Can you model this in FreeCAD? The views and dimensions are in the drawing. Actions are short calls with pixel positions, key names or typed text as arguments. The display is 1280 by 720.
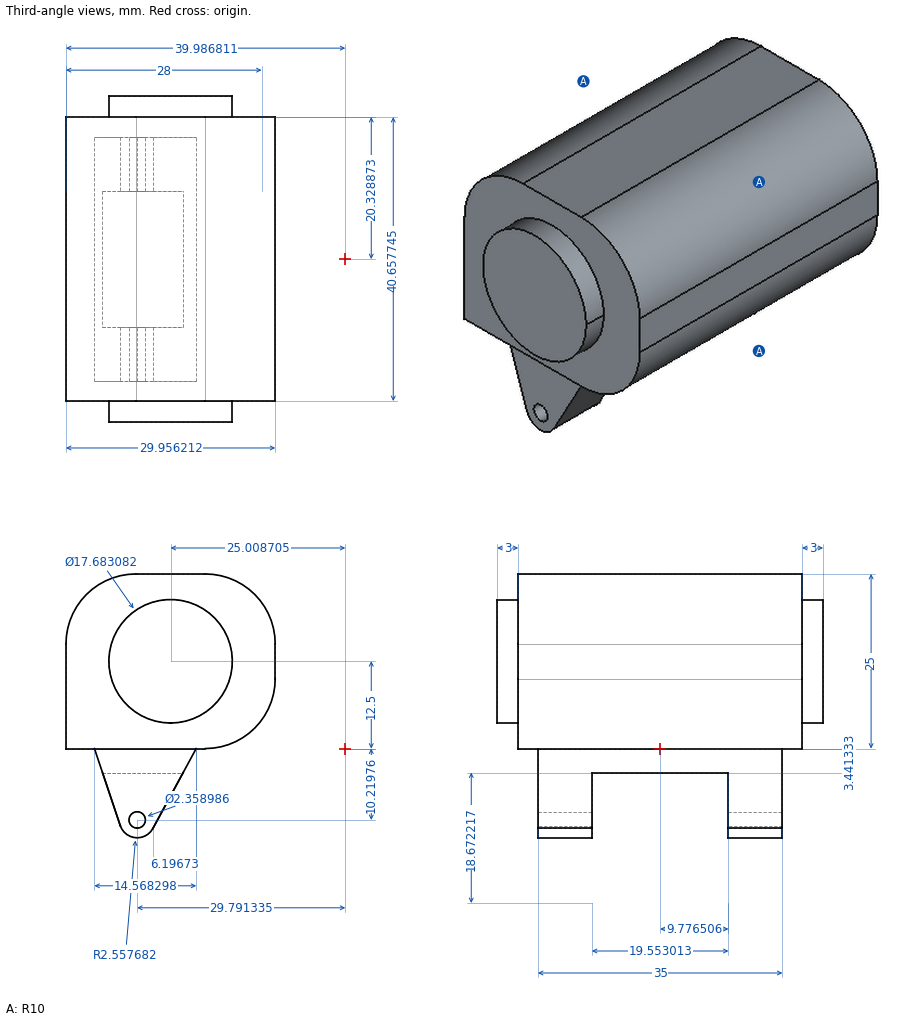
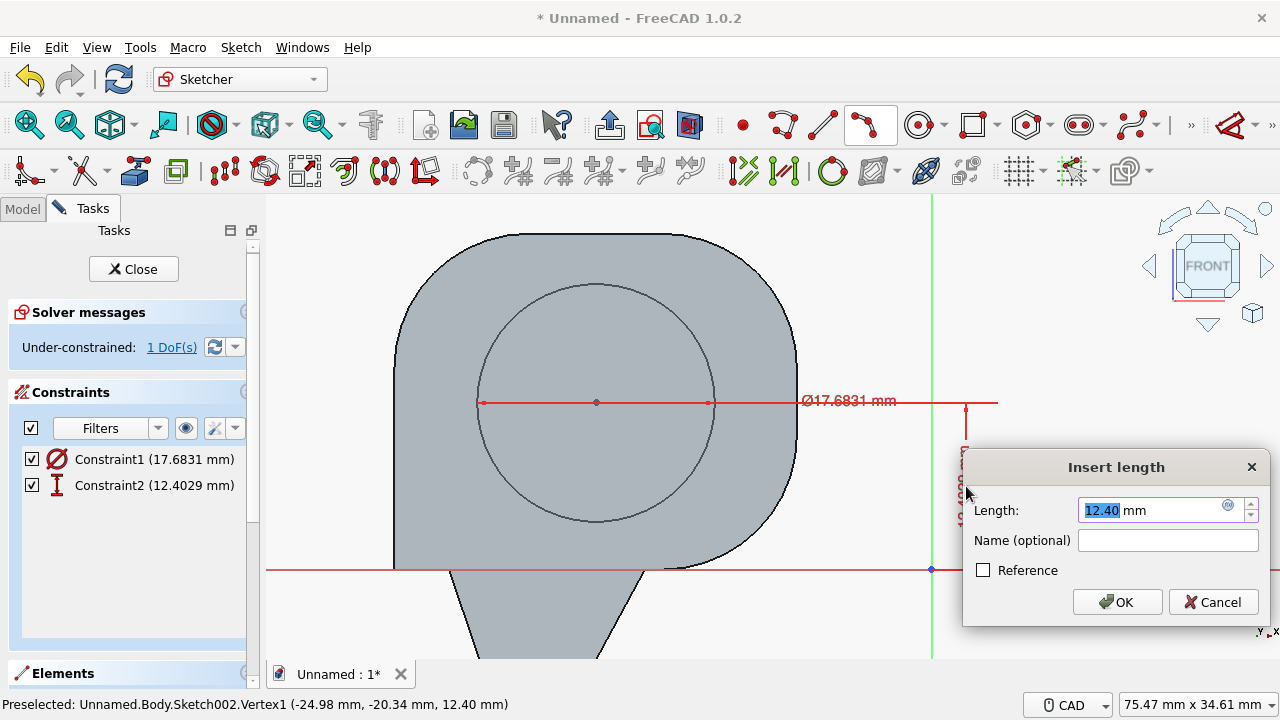
text(12.5)
key(Return)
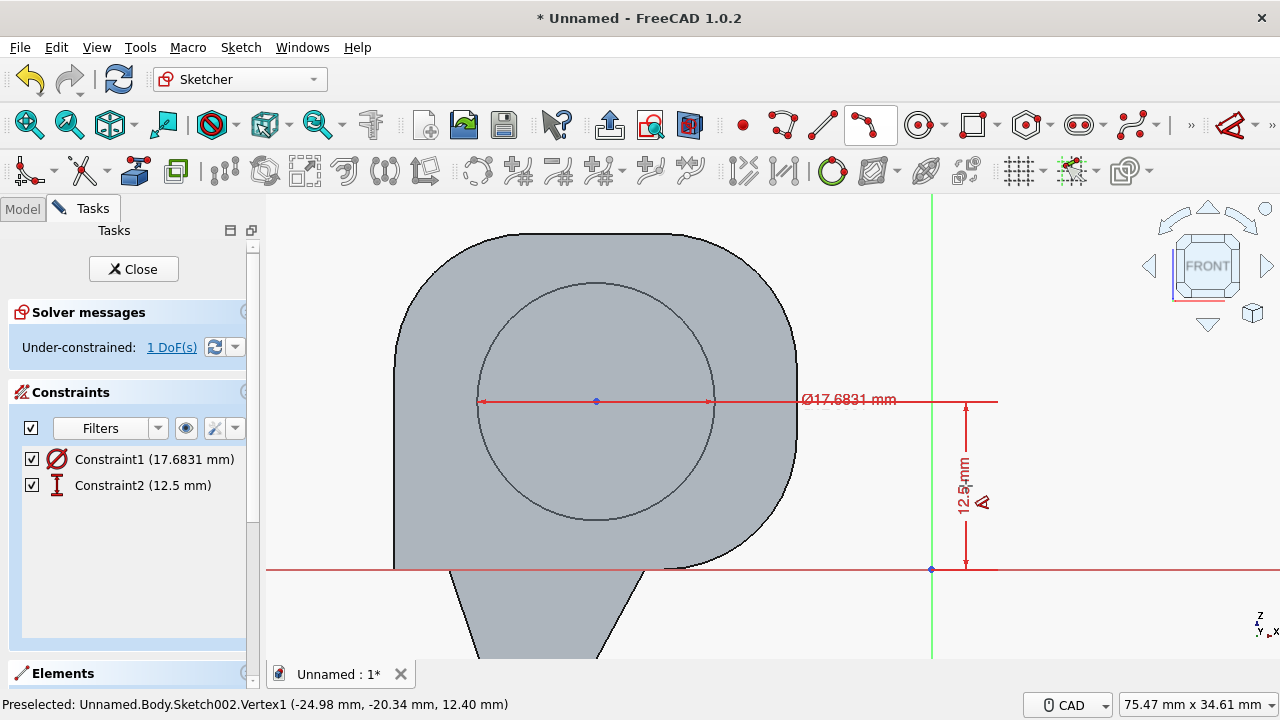
click(596, 402)
click(764, 604)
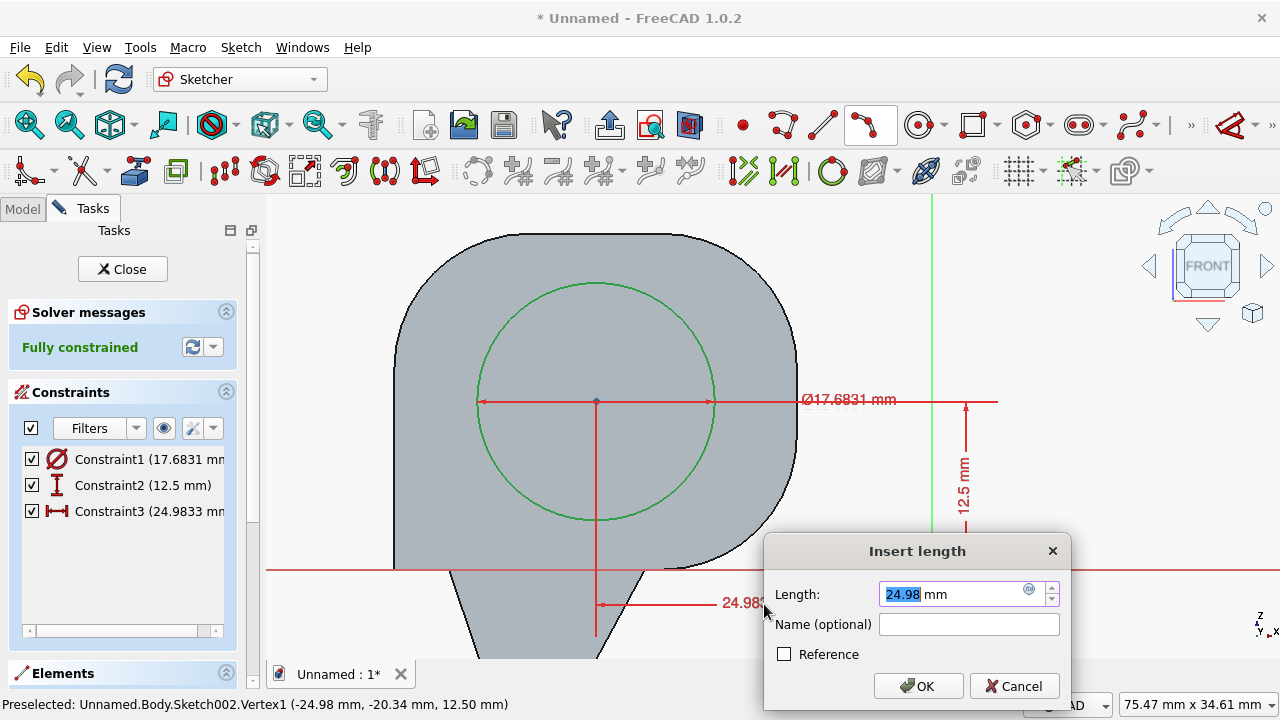
text(25.008705)
key(Return)
key(Escape)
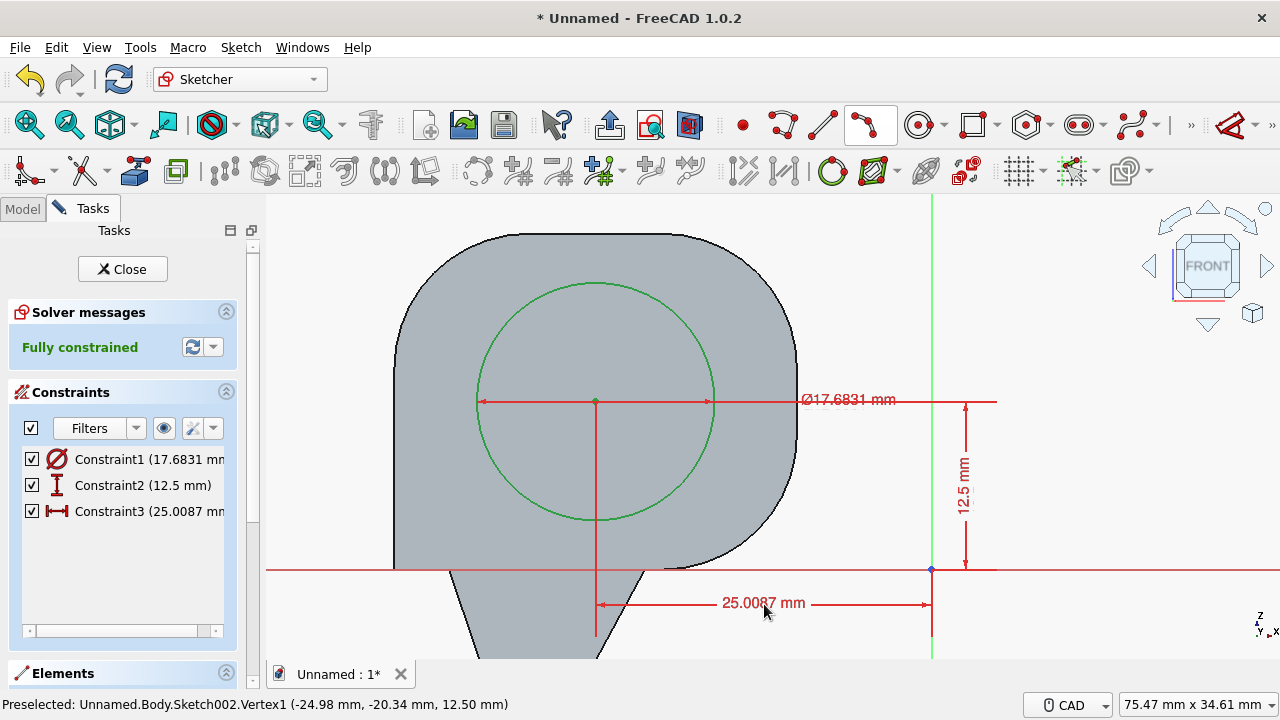
click(123, 269)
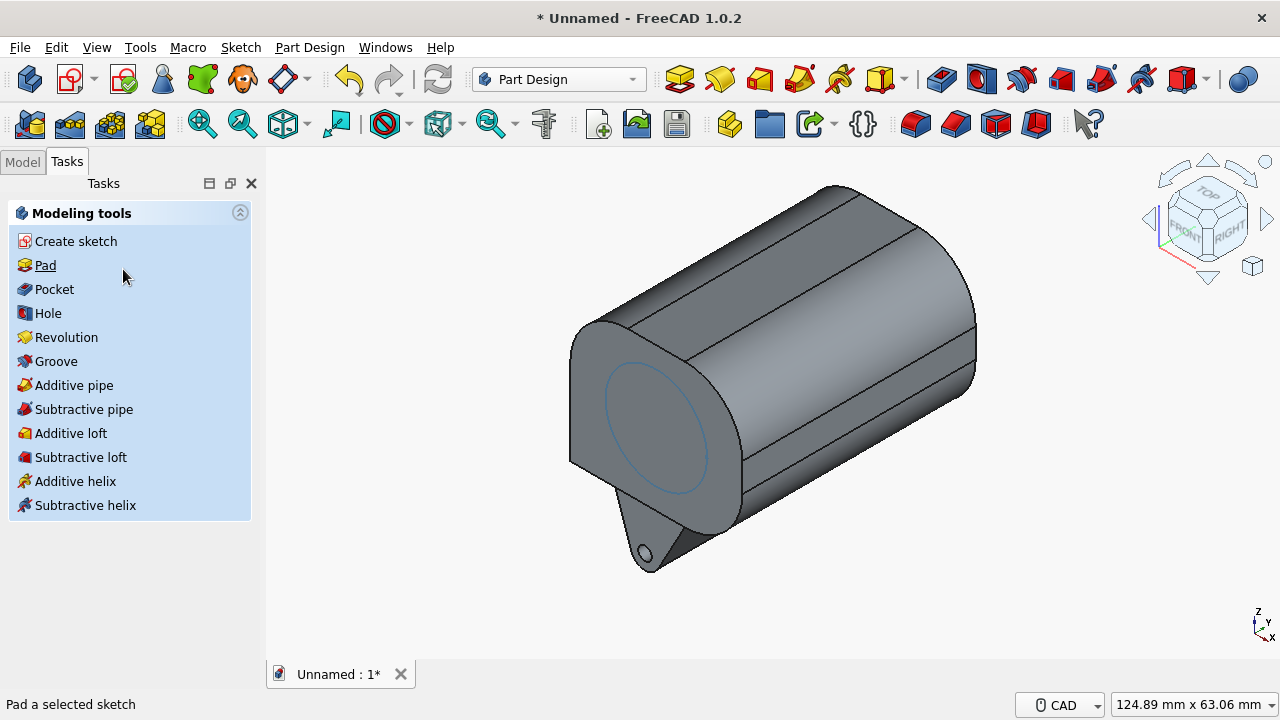
click(680, 80)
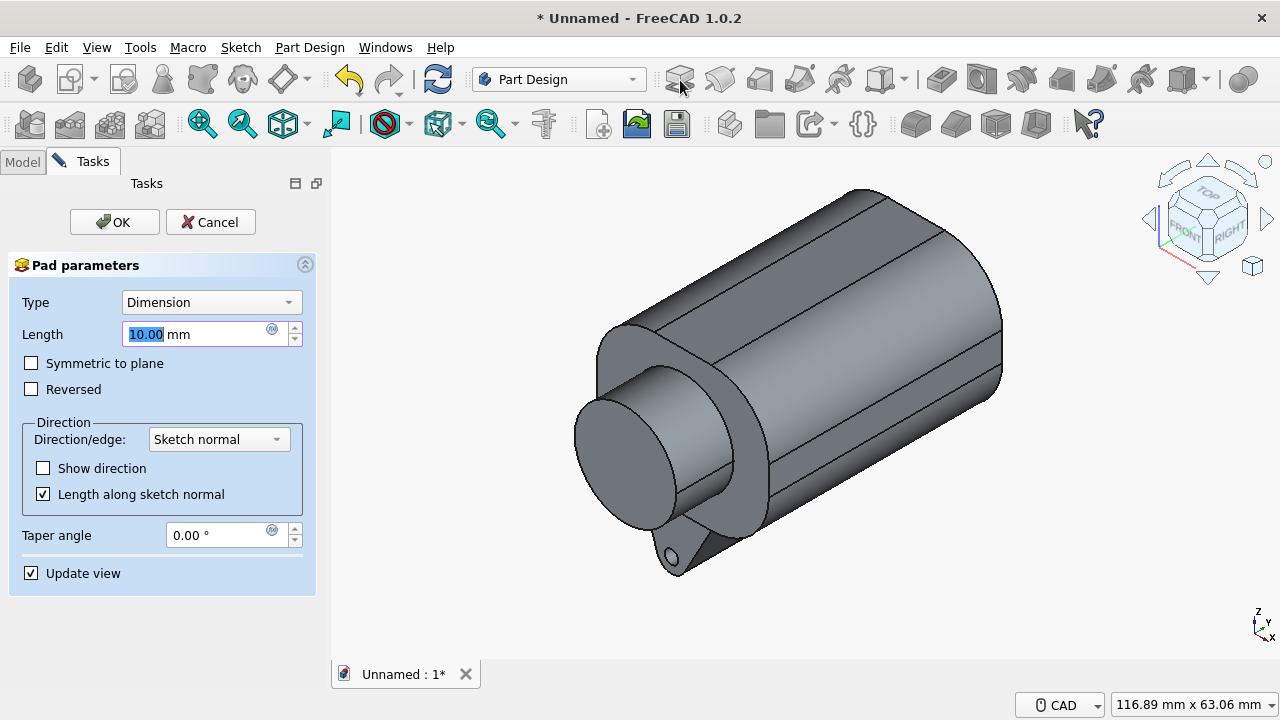
text(3)
key(Tab)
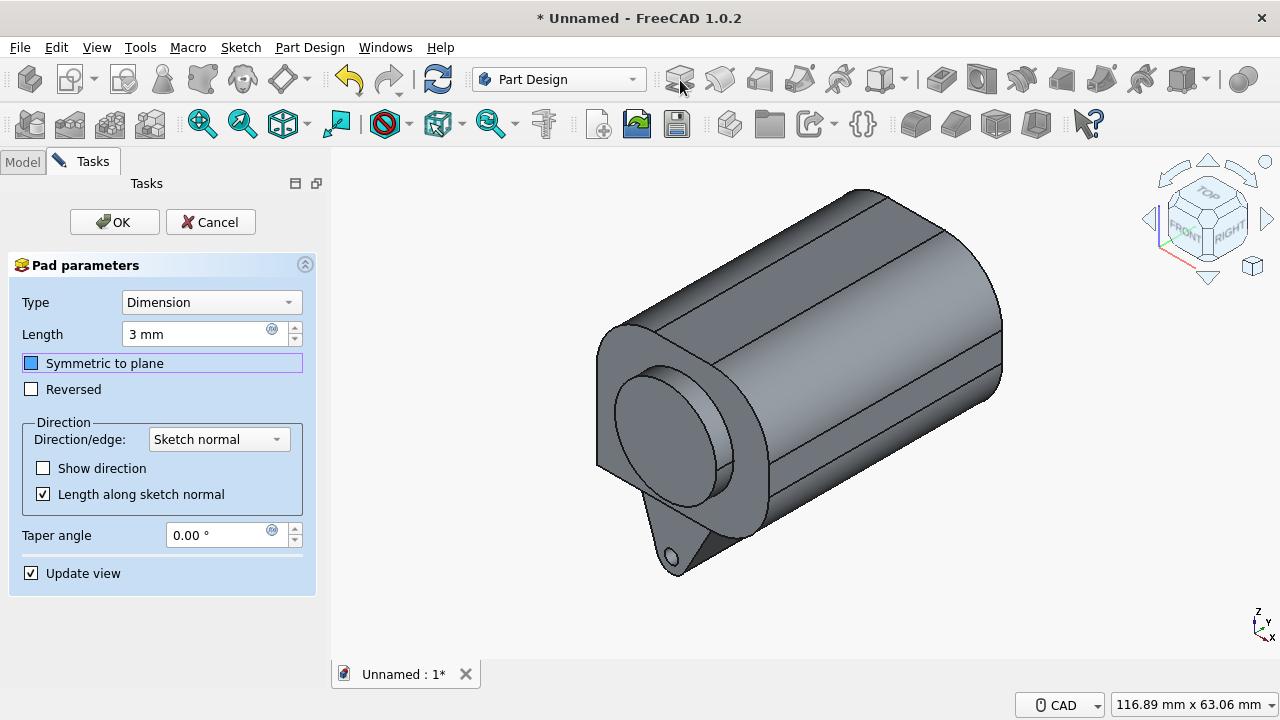
click(115, 222)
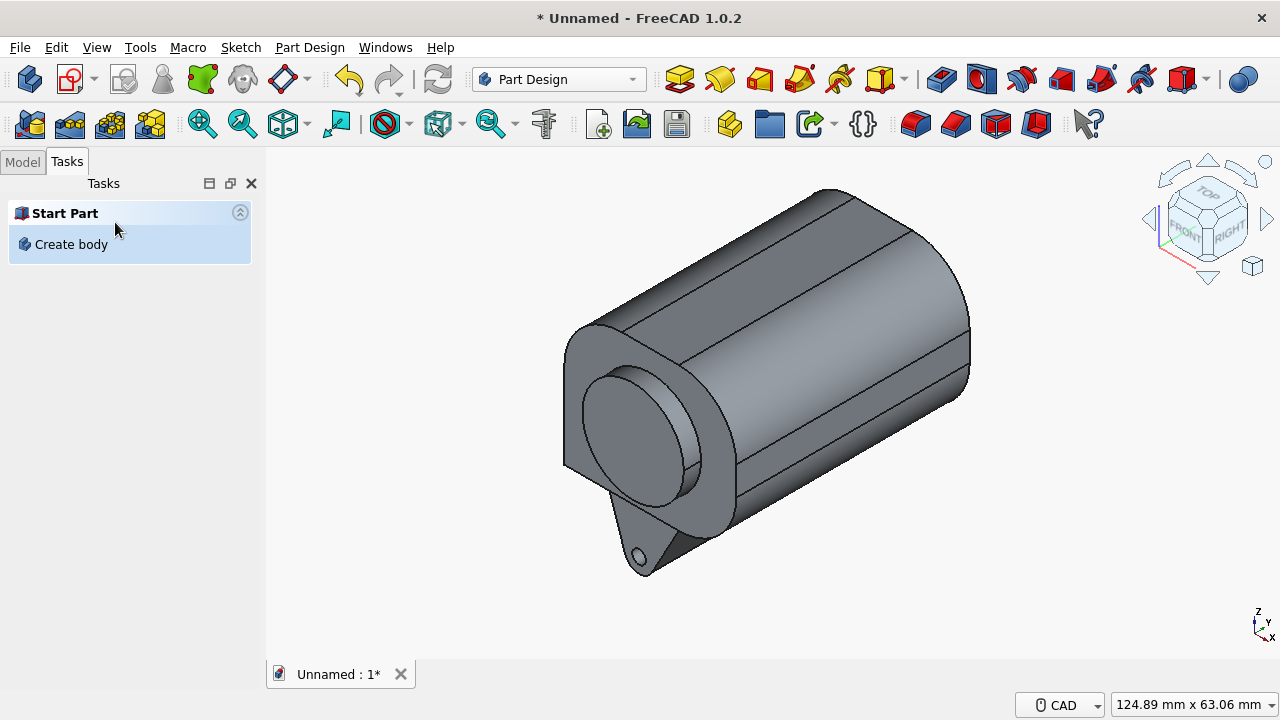
click(23, 161)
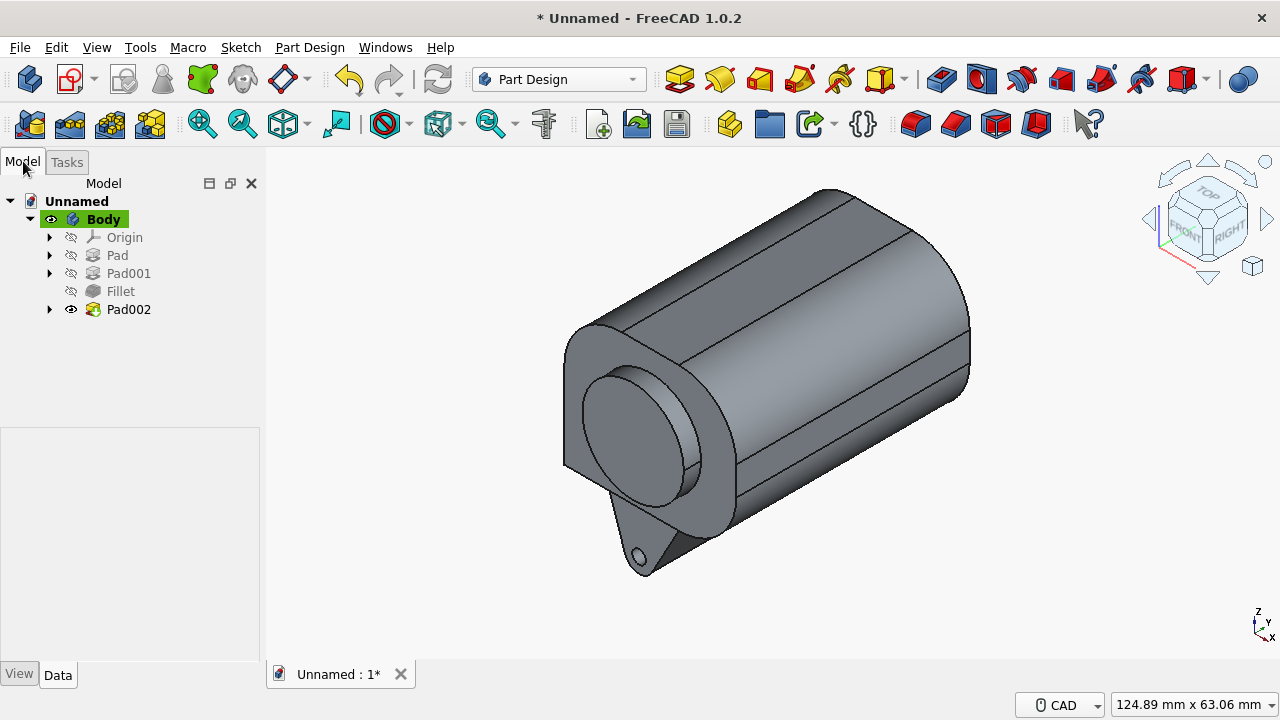
click(50, 237)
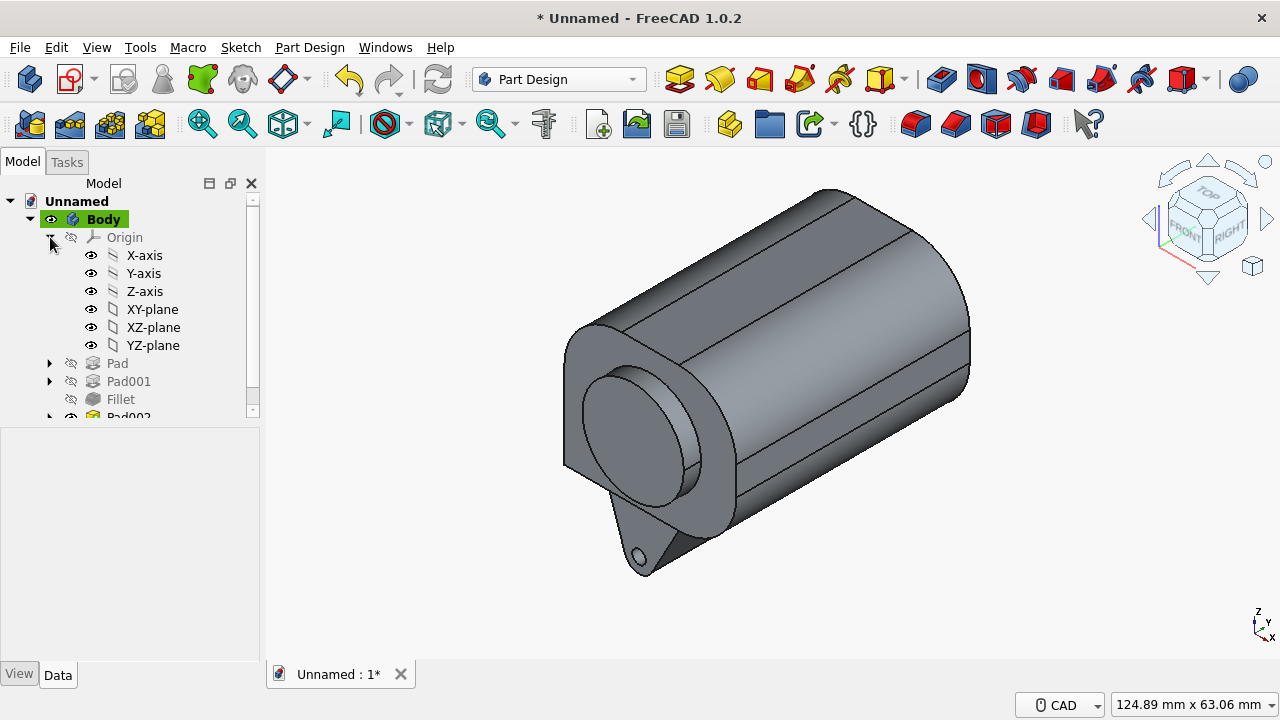
click(136, 327)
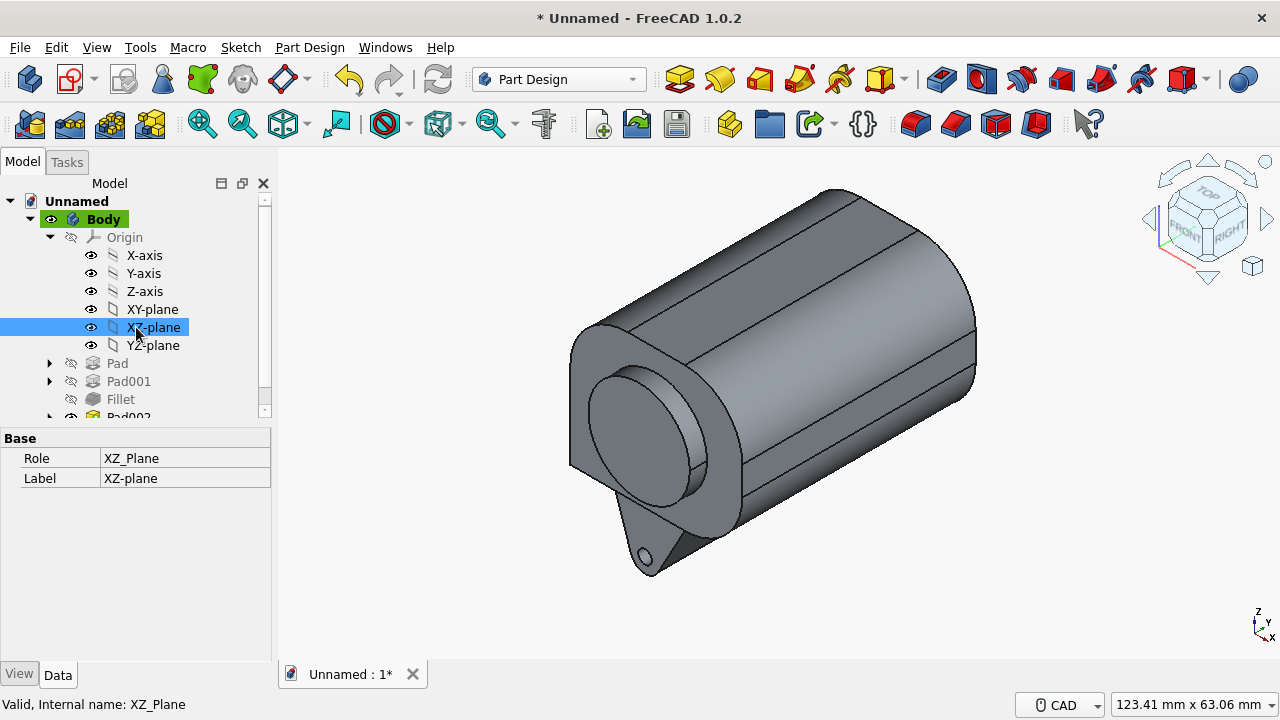
click(284, 80)